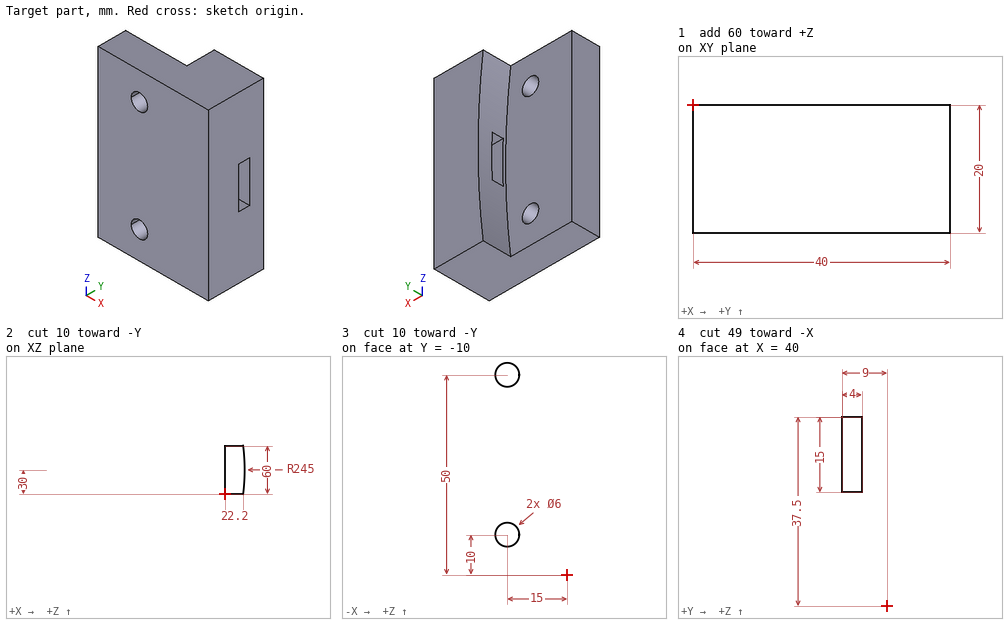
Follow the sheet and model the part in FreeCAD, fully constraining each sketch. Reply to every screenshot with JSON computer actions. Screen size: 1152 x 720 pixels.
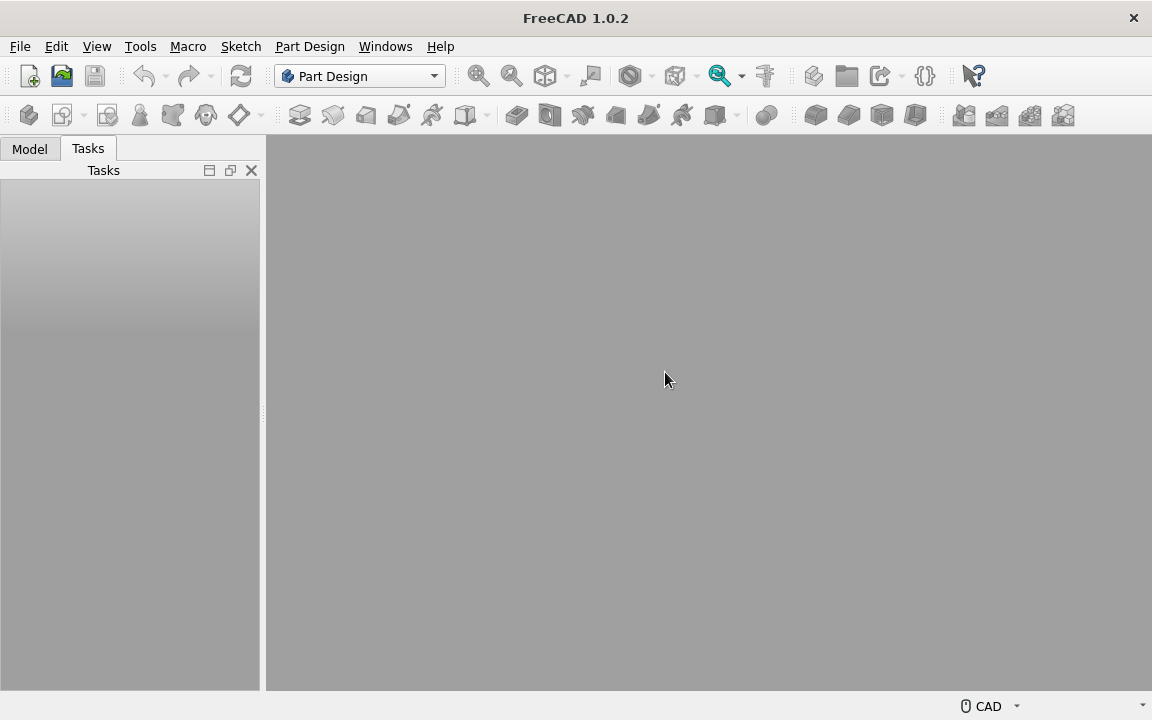
{"action": "left_click", "coordinate": [29, 76]}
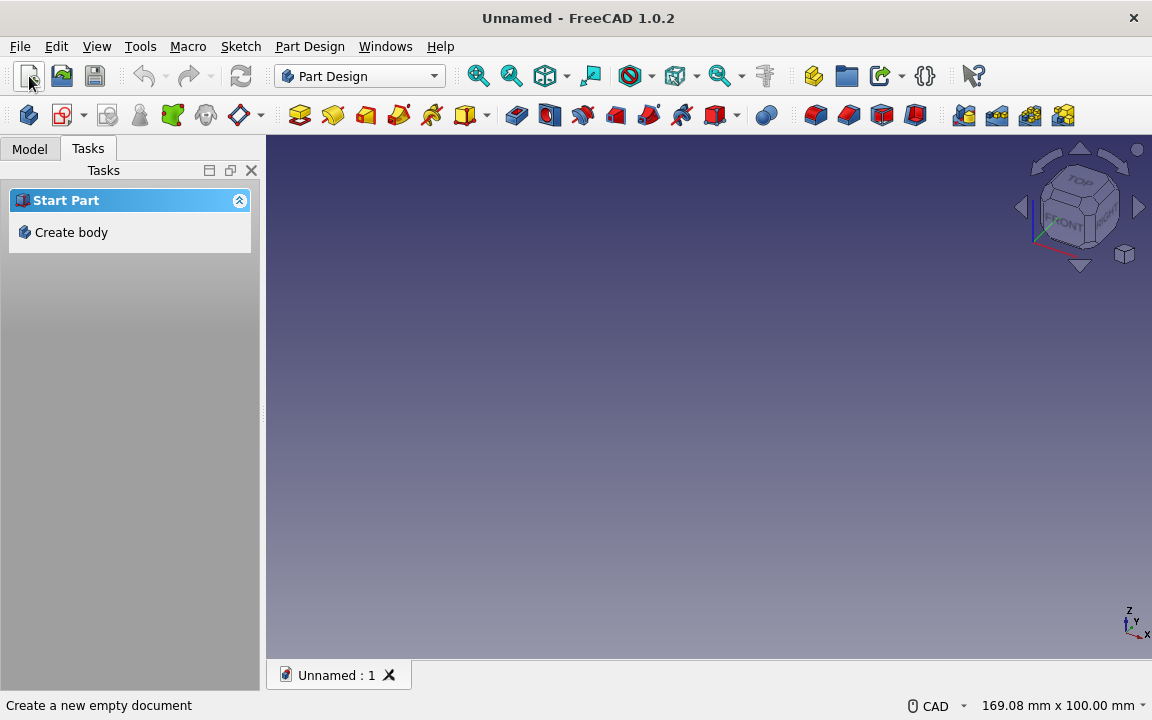
{"action": "left_click", "coordinate": [62, 116]}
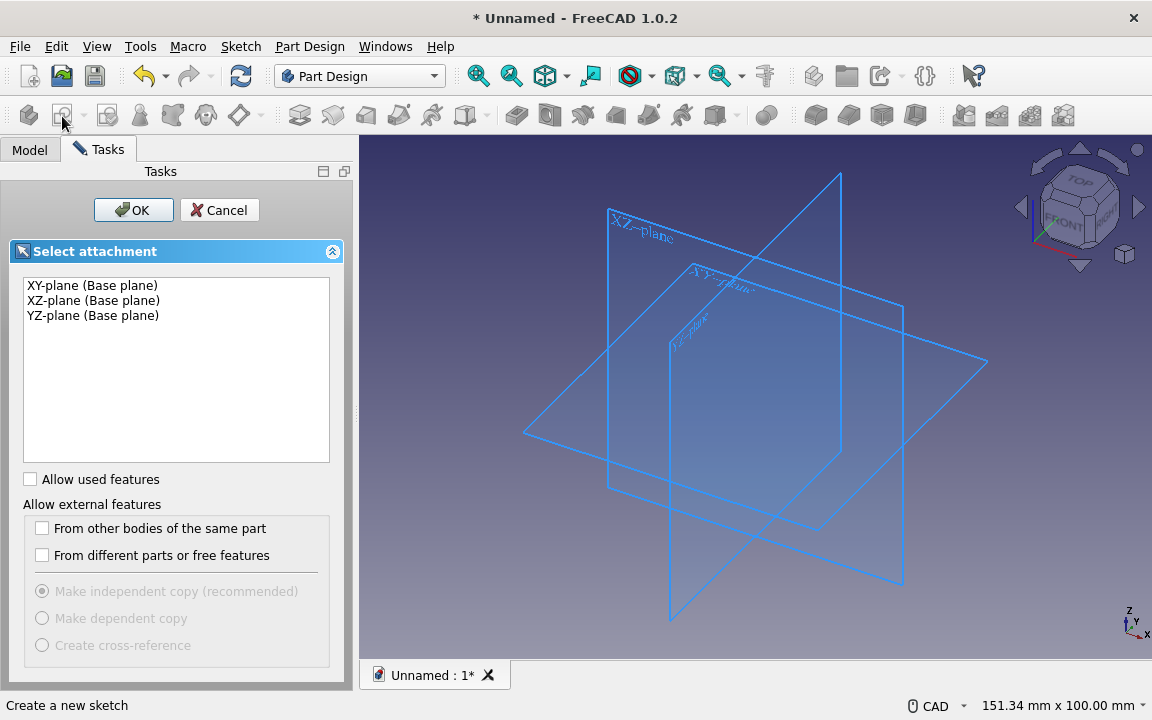
{"action": "left_click", "coordinate": [84, 286]}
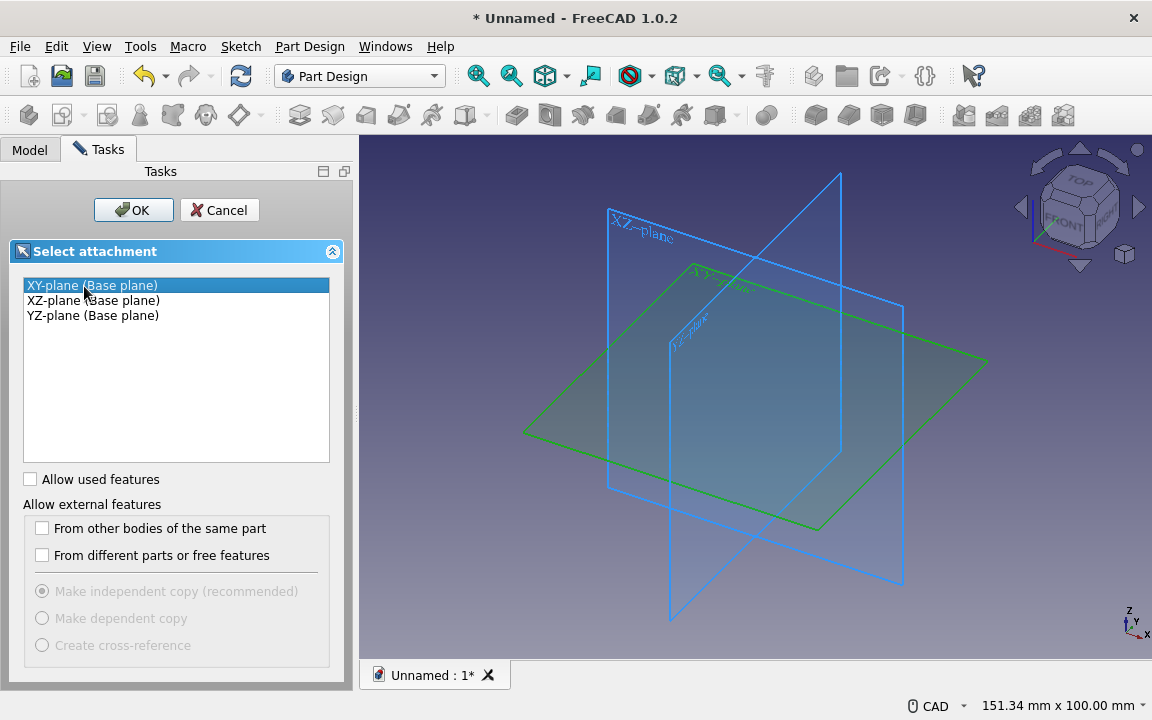
{"action": "left_click", "coordinate": [134, 210]}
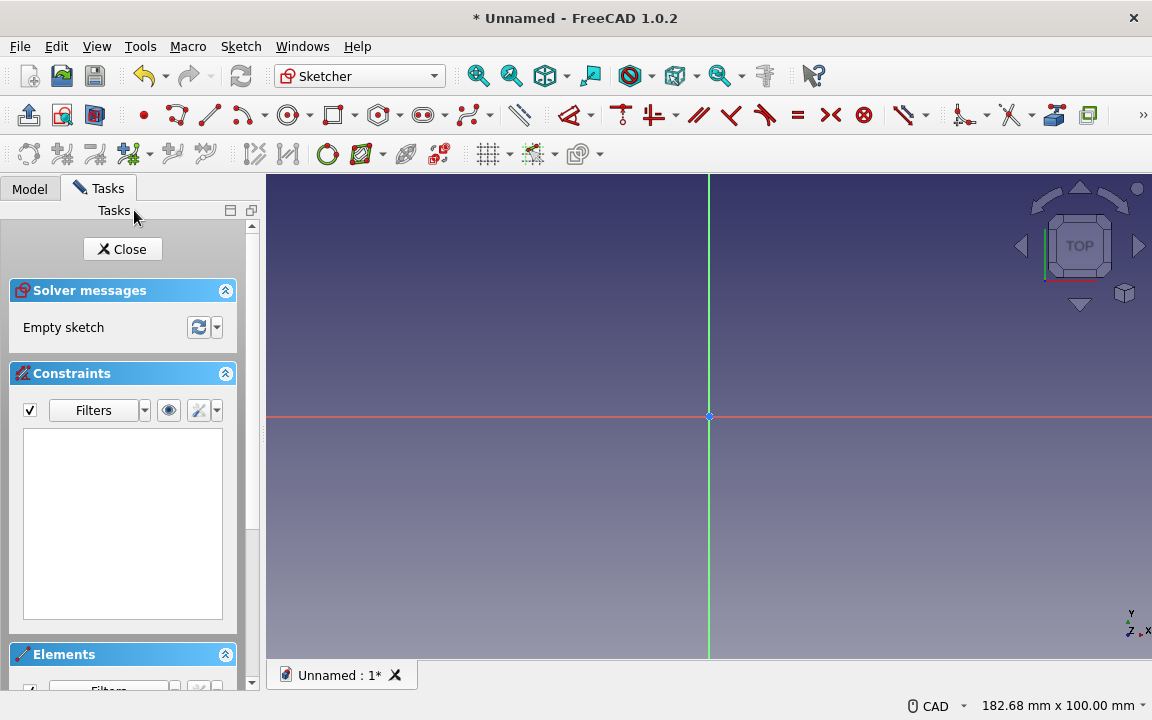
{"action": "scroll", "coordinate": [902, 493], "scroll_direction": "up", "scroll_amount": 5}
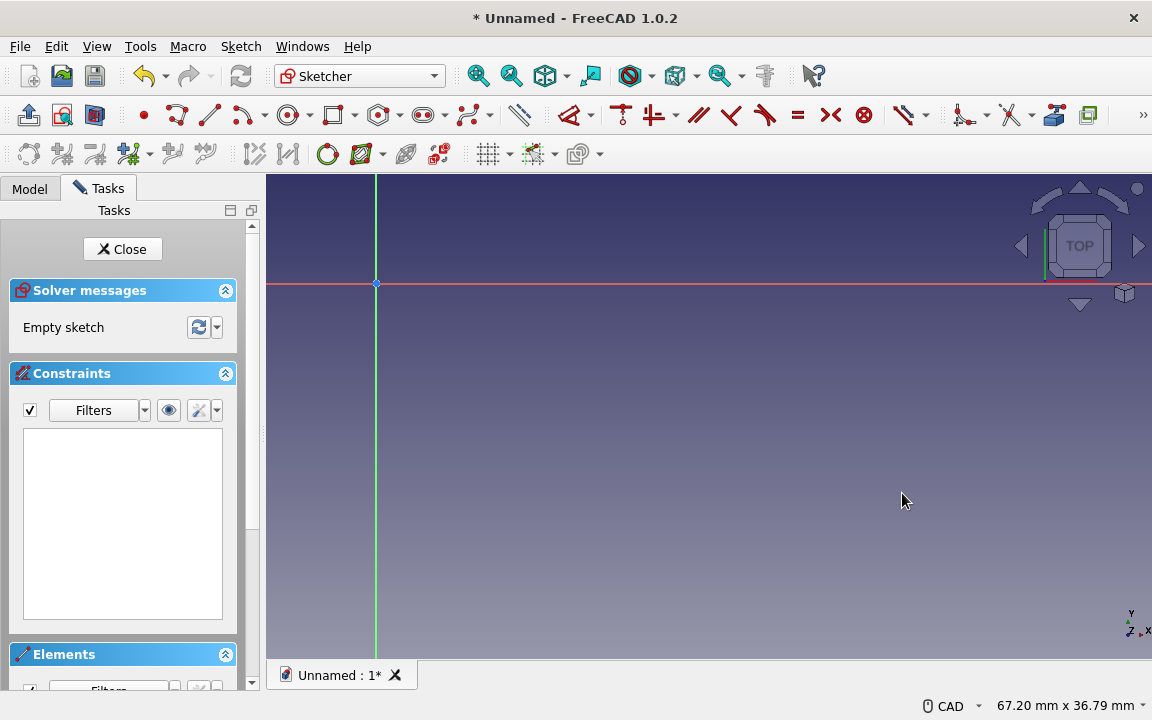
{"action": "left_click", "coordinate": [332, 116]}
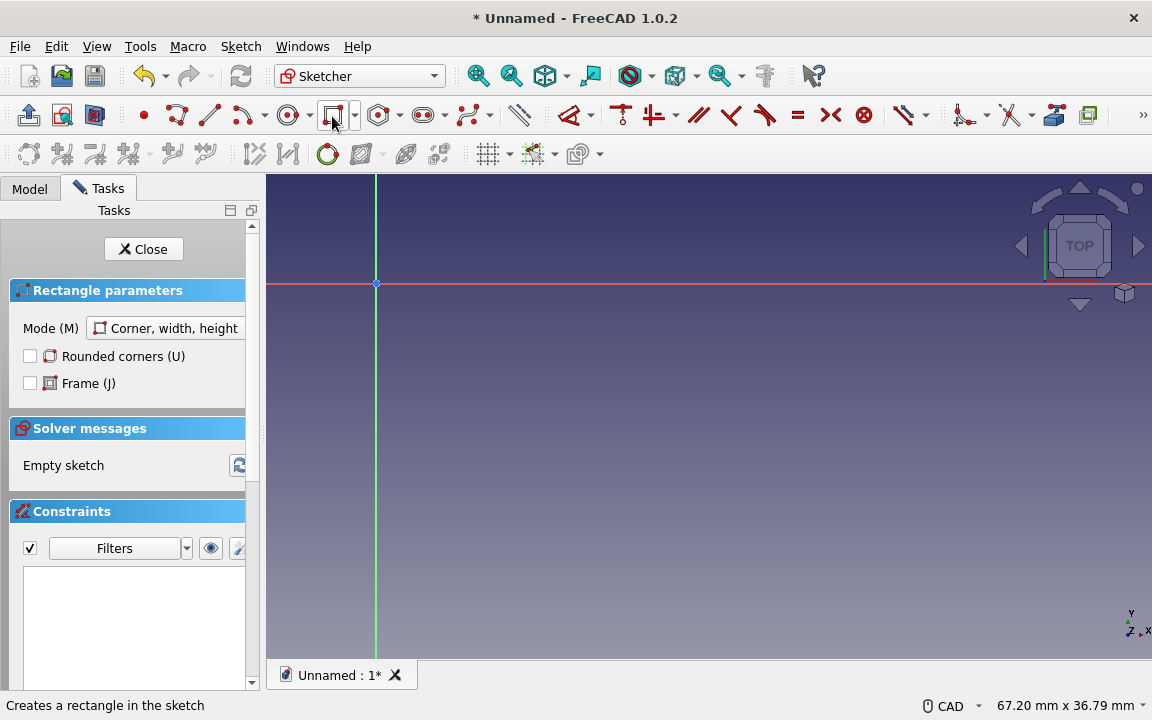
{"action": "left_click", "coordinate": [376, 284]}
{"action": "mouse_move", "coordinate": [903, 548]}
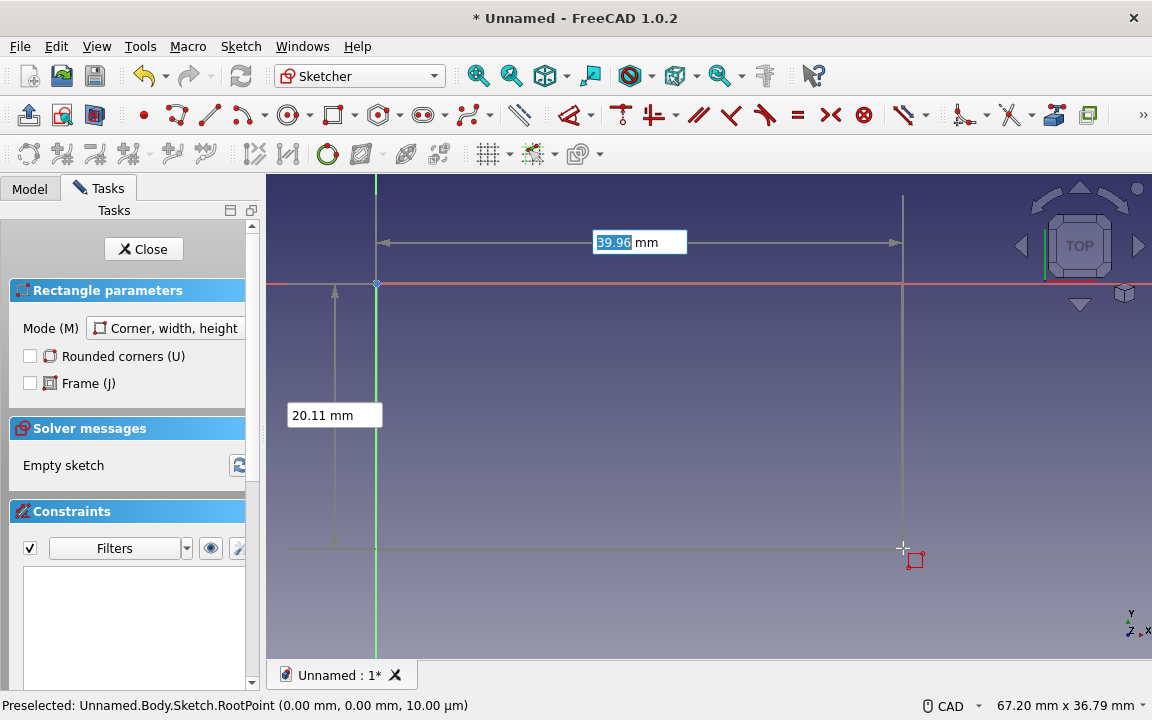
{"action": "type", "text": "40"}
{"action": "key", "text": "Tab"}
{"action": "type", "text": "20"}
{"action": "key", "text": "Return"}
{"action": "key", "text": "Escape"}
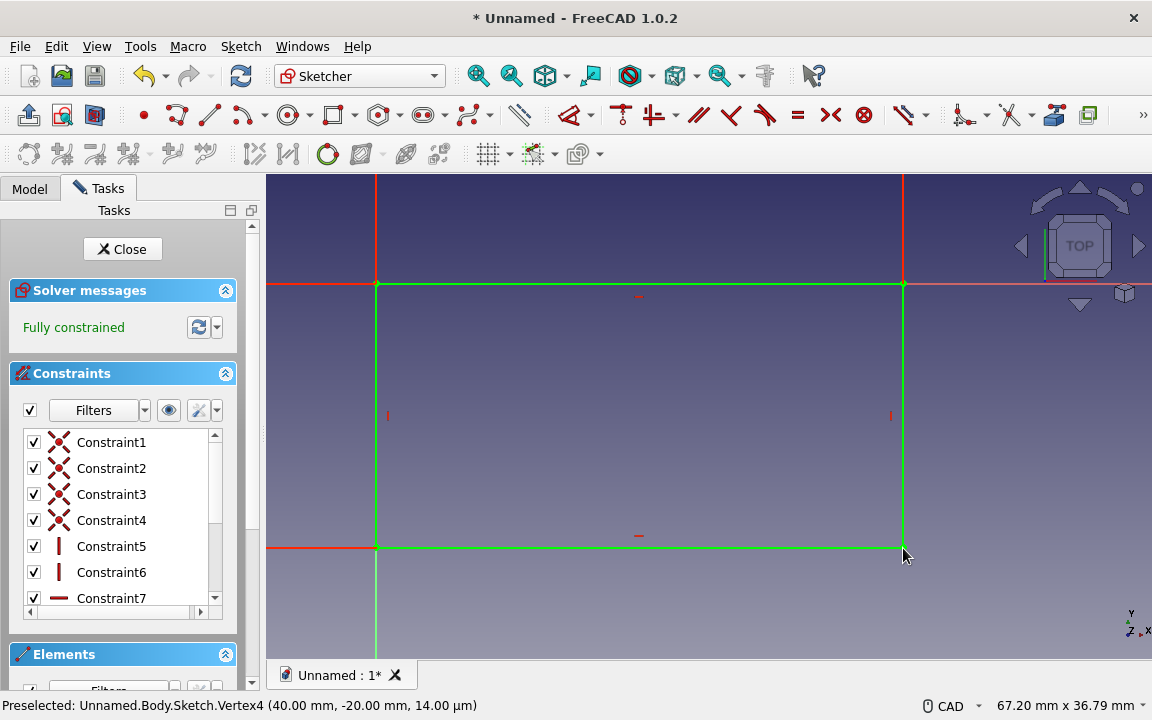
{"action": "left_click", "coordinate": [123, 249]}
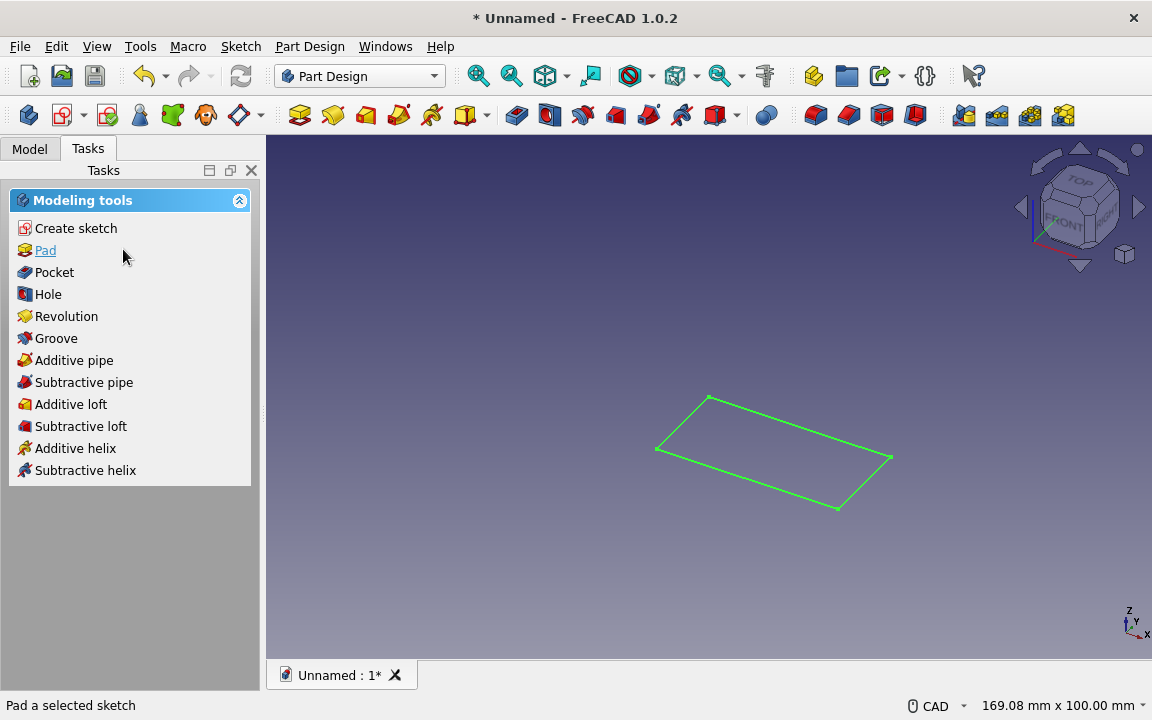
{"action": "left_click", "coordinate": [300, 116]}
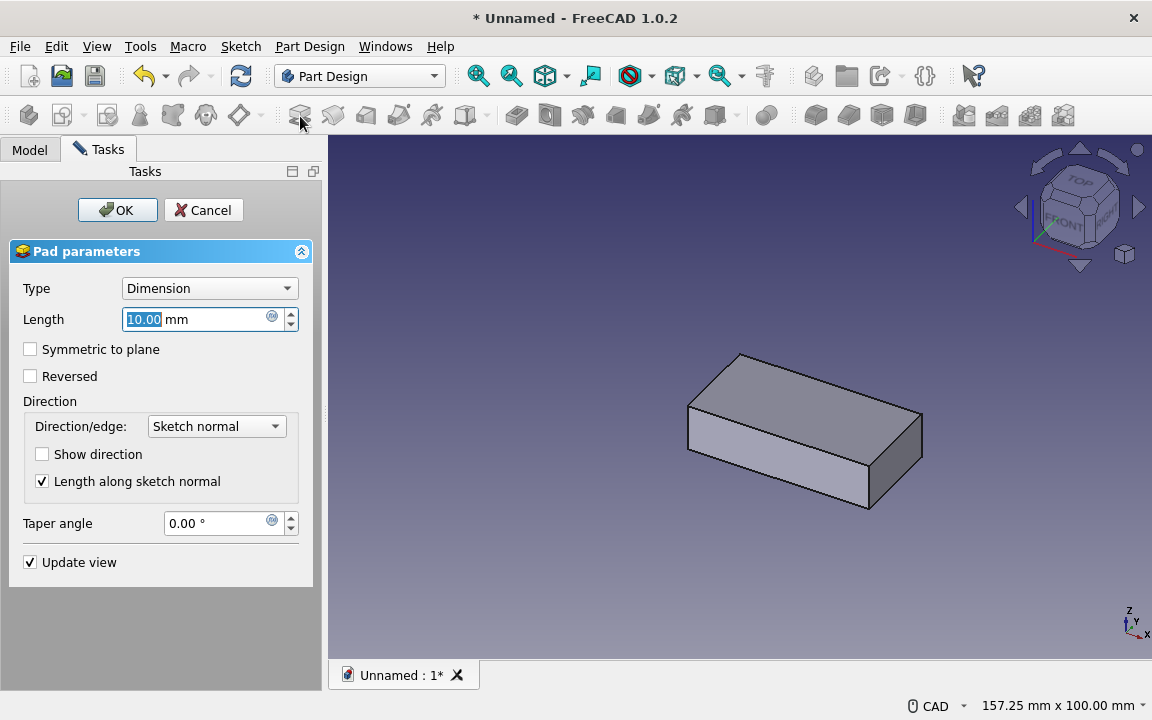
{"action": "type", "text": "60"}
{"action": "key", "text": "Tab"}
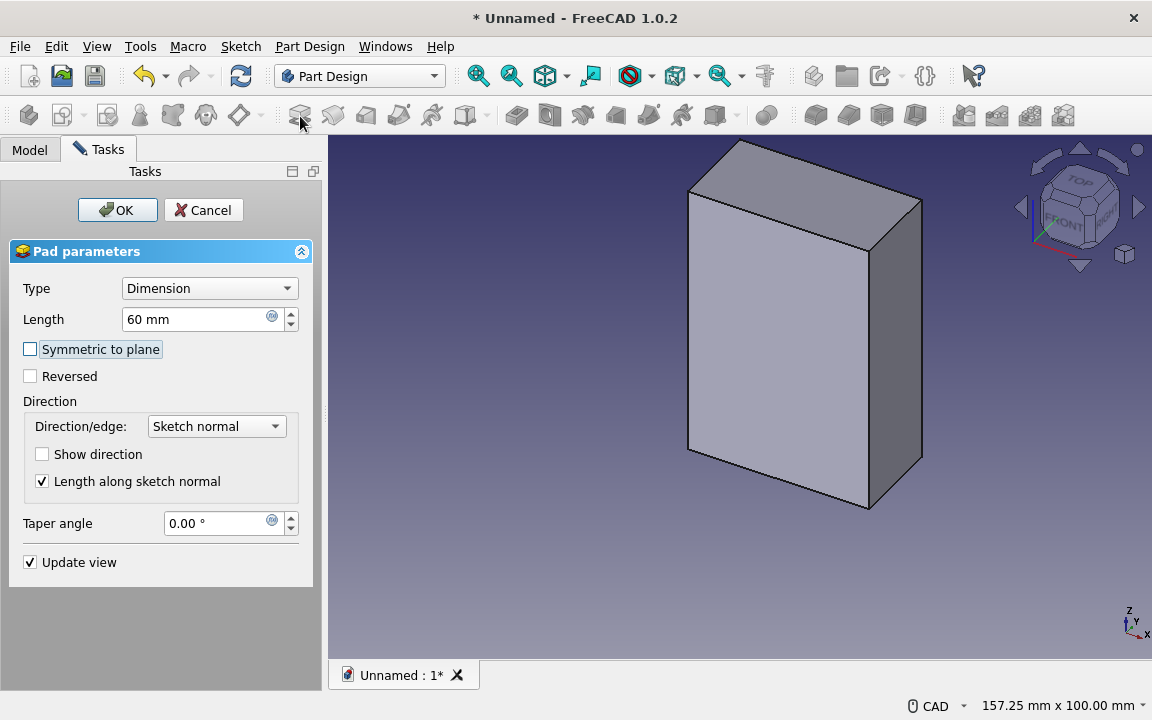
{"action": "left_click", "coordinate": [118, 210]}